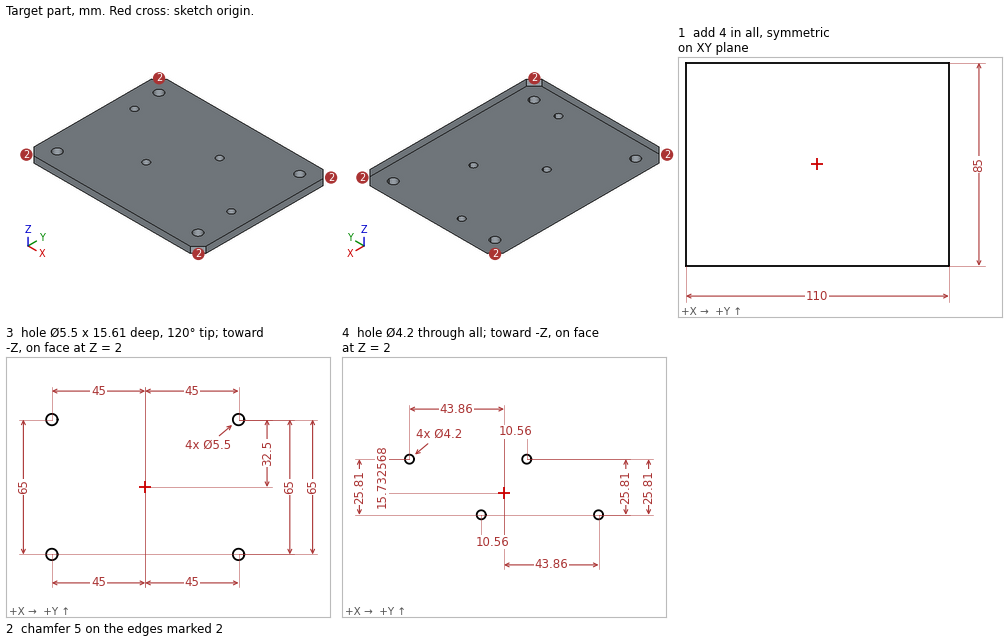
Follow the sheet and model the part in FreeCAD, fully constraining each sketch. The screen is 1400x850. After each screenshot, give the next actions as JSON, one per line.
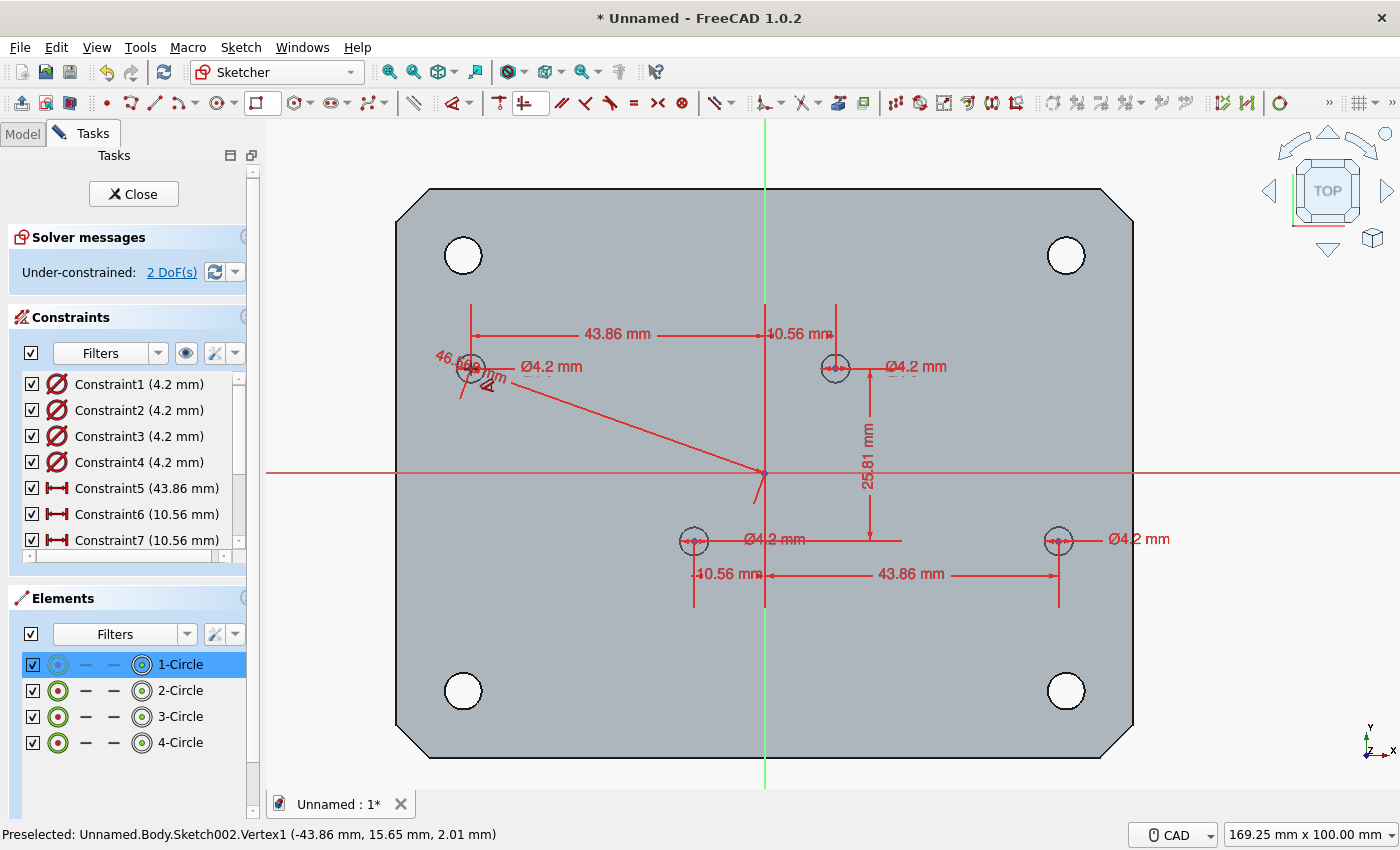
{"action": "left_click", "coordinate": [694, 541]}
{"action": "left_click", "coordinate": [437, 455]}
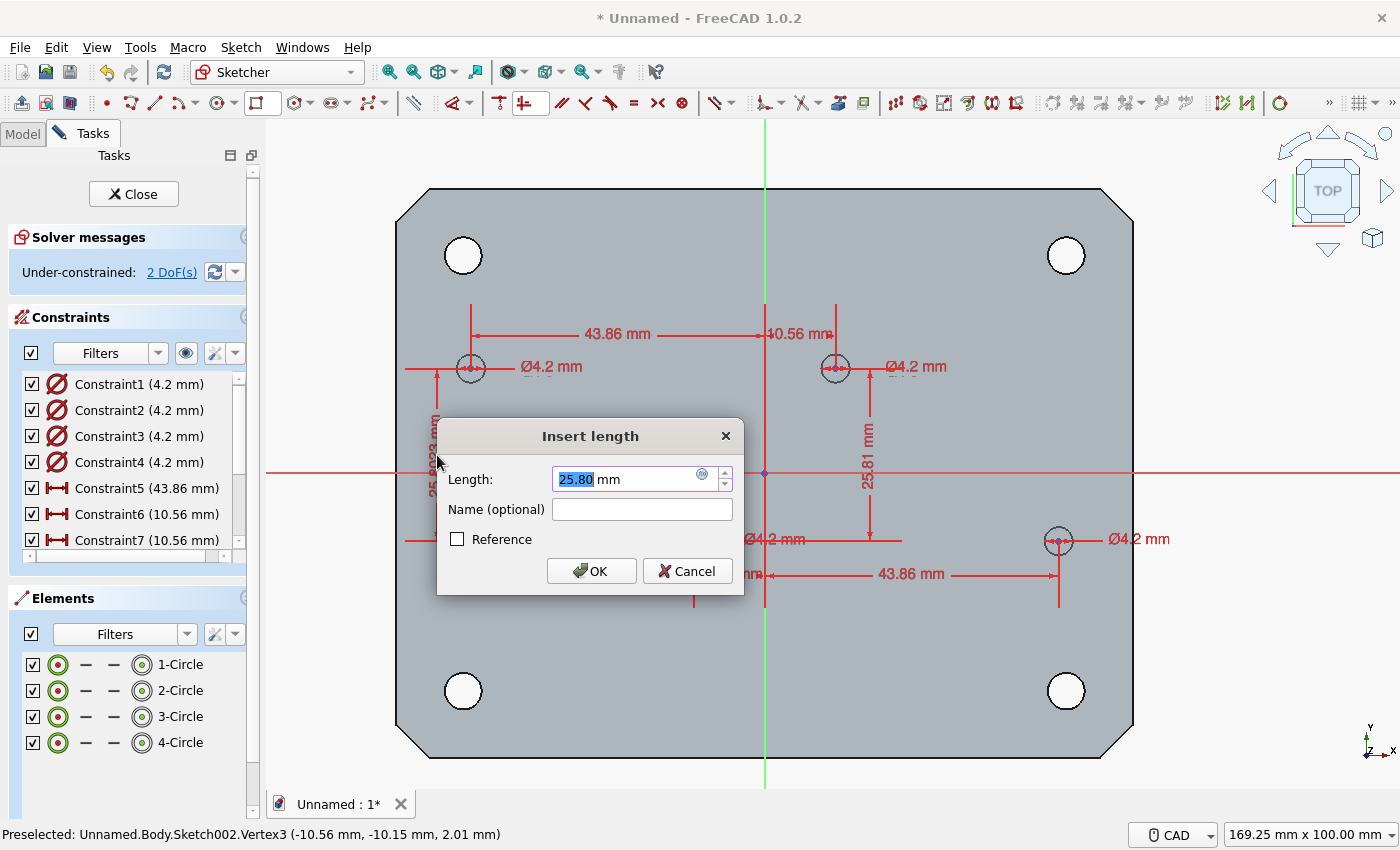
{"action": "type", "text": "25.81"}
{"action": "key", "text": "Return"}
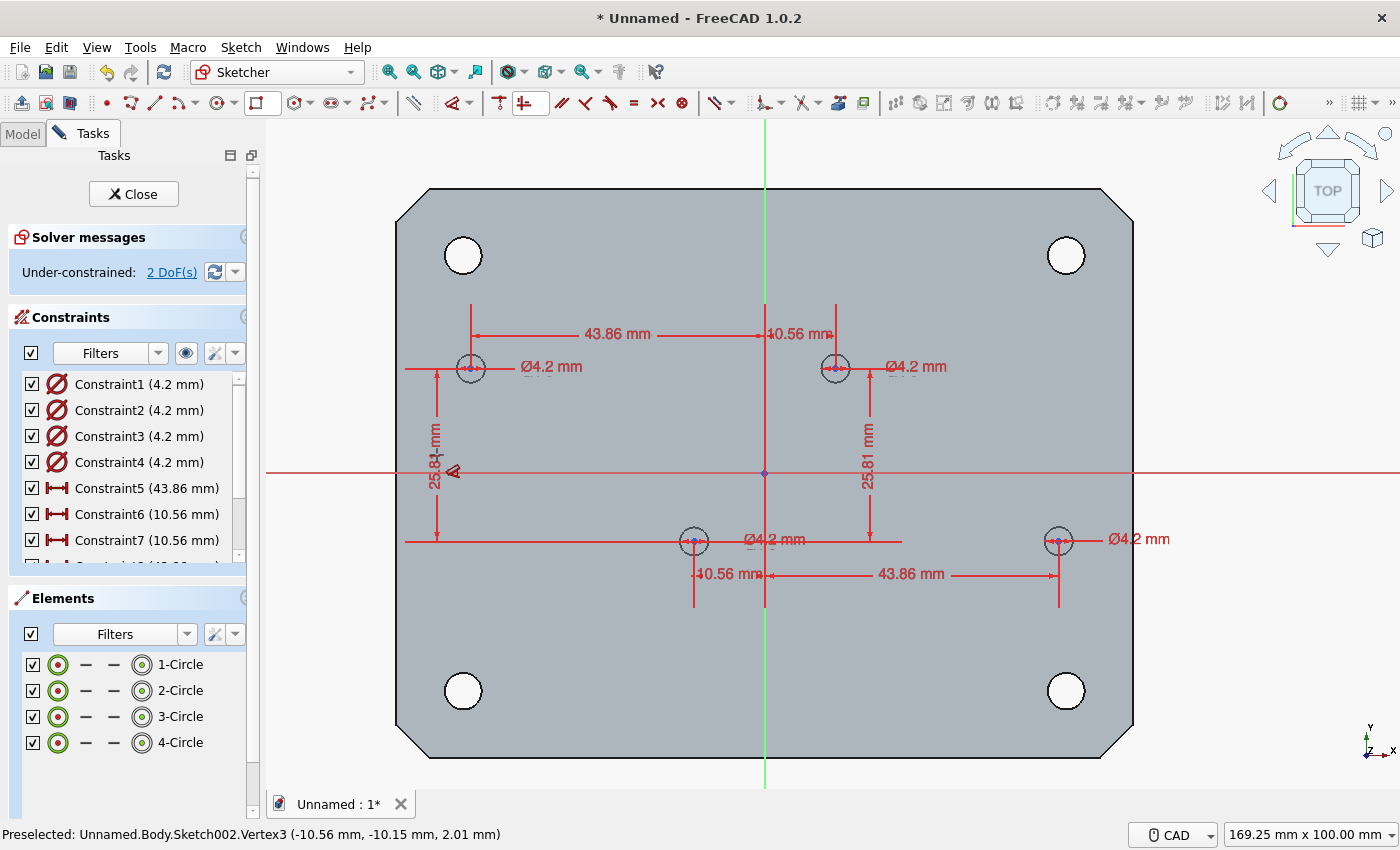
{"action": "left_click", "coordinate": [836, 369]}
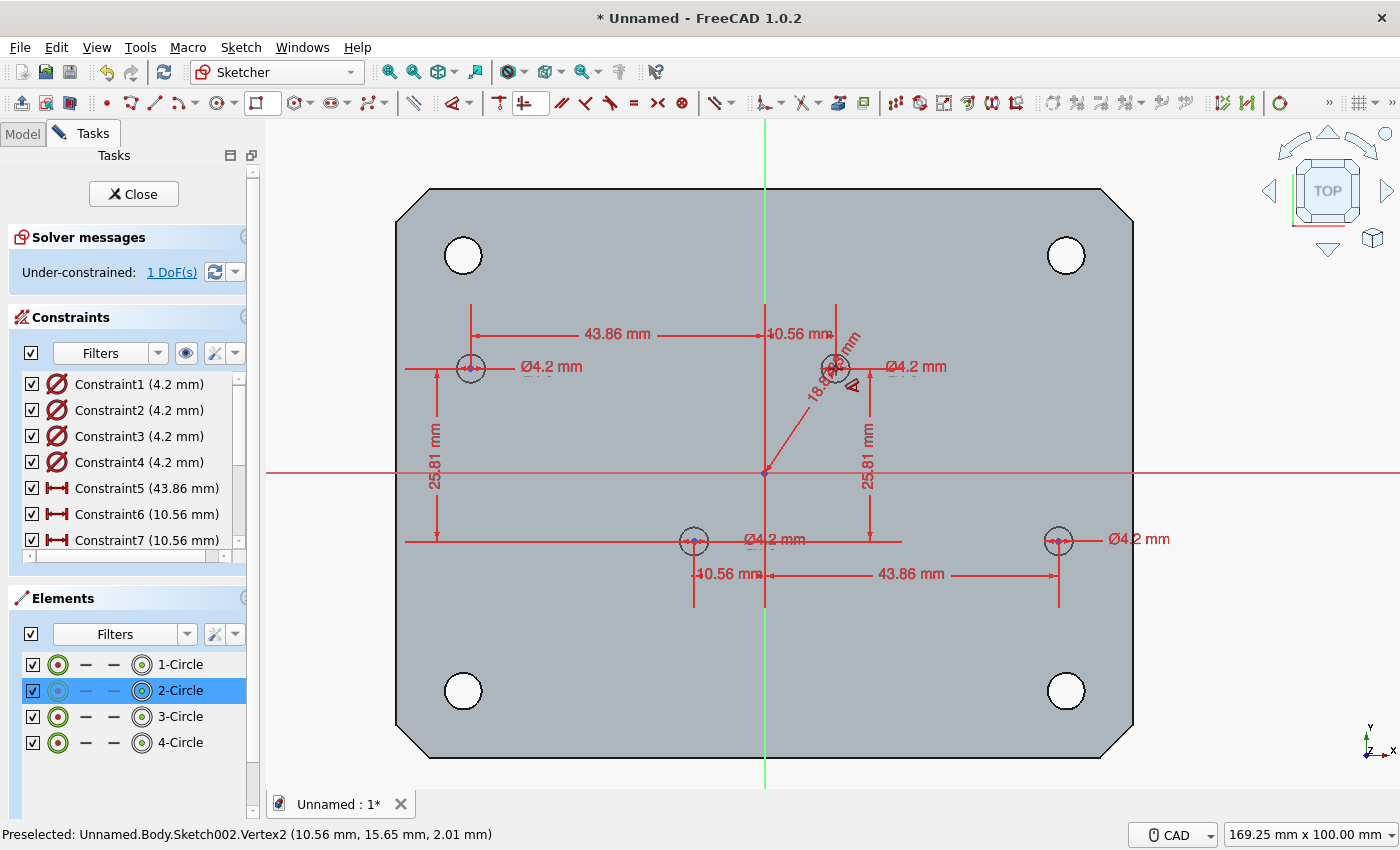
{"action": "left_click", "coordinate": [1059, 541]}
{"action": "left_click", "coordinate": [1093, 455]}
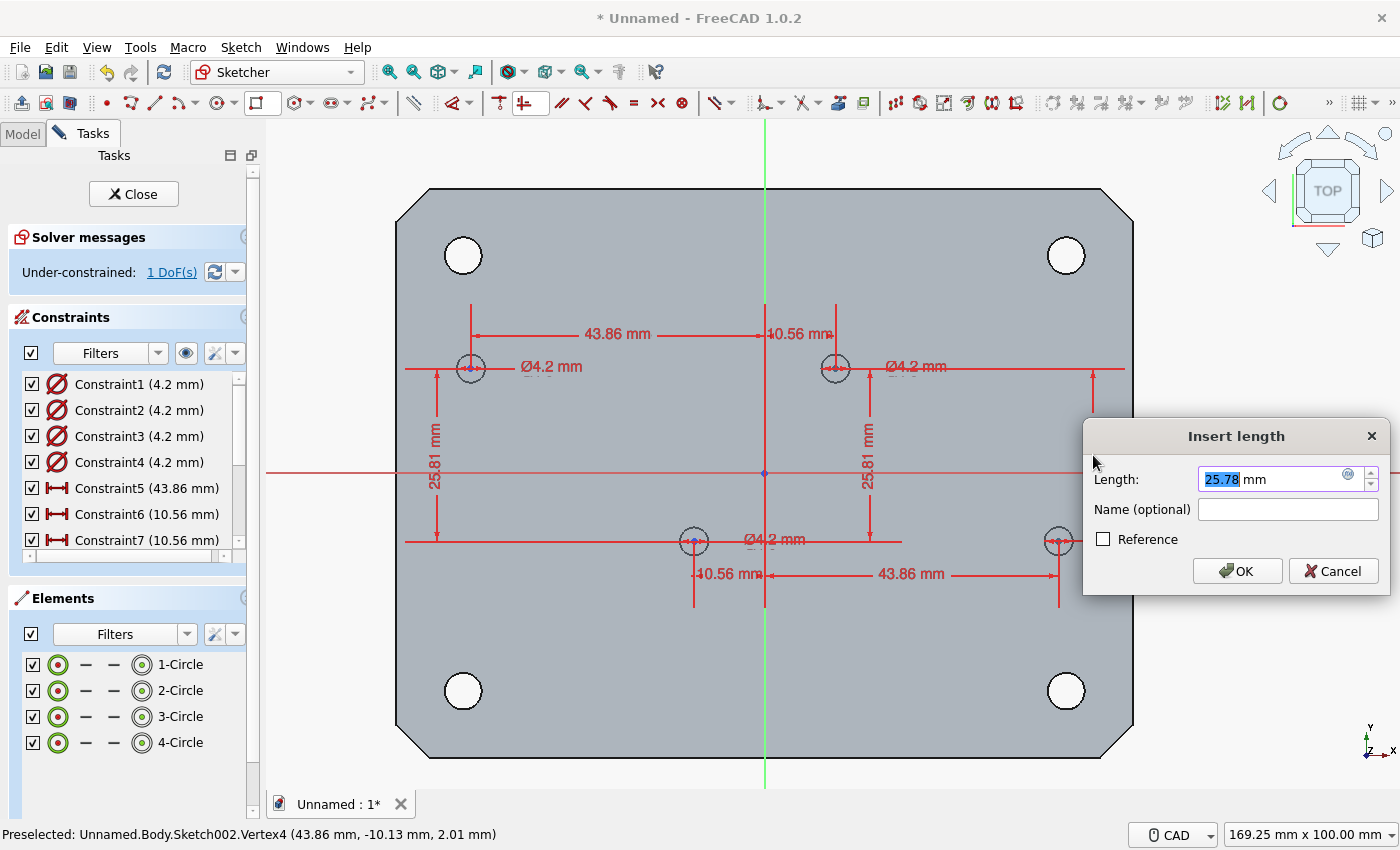
{"action": "type", "text": "25.81"}
{"action": "key", "text": "Return"}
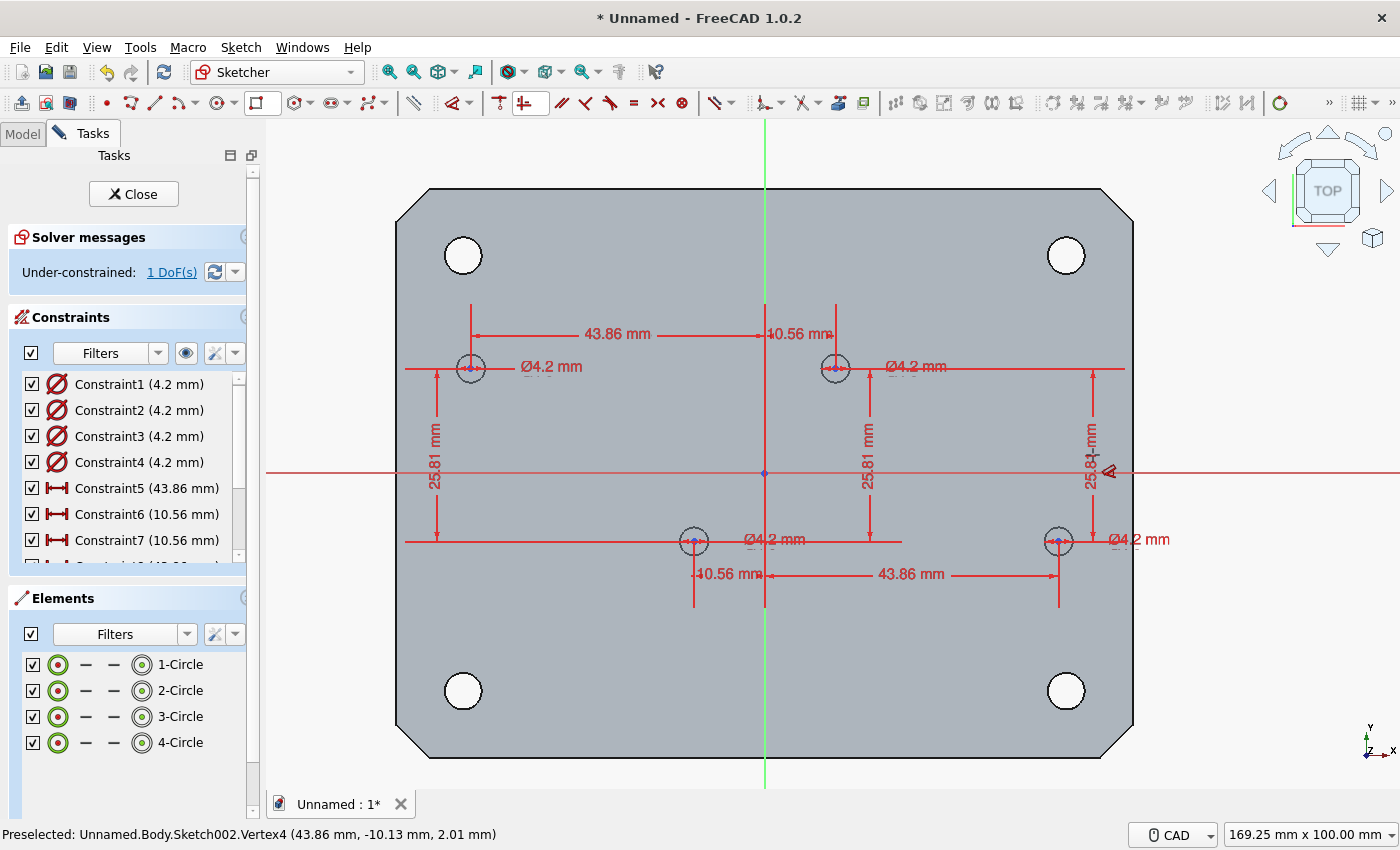
{"action": "left_click", "coordinate": [471, 369]}
{"action": "left_click", "coordinate": [437, 421]}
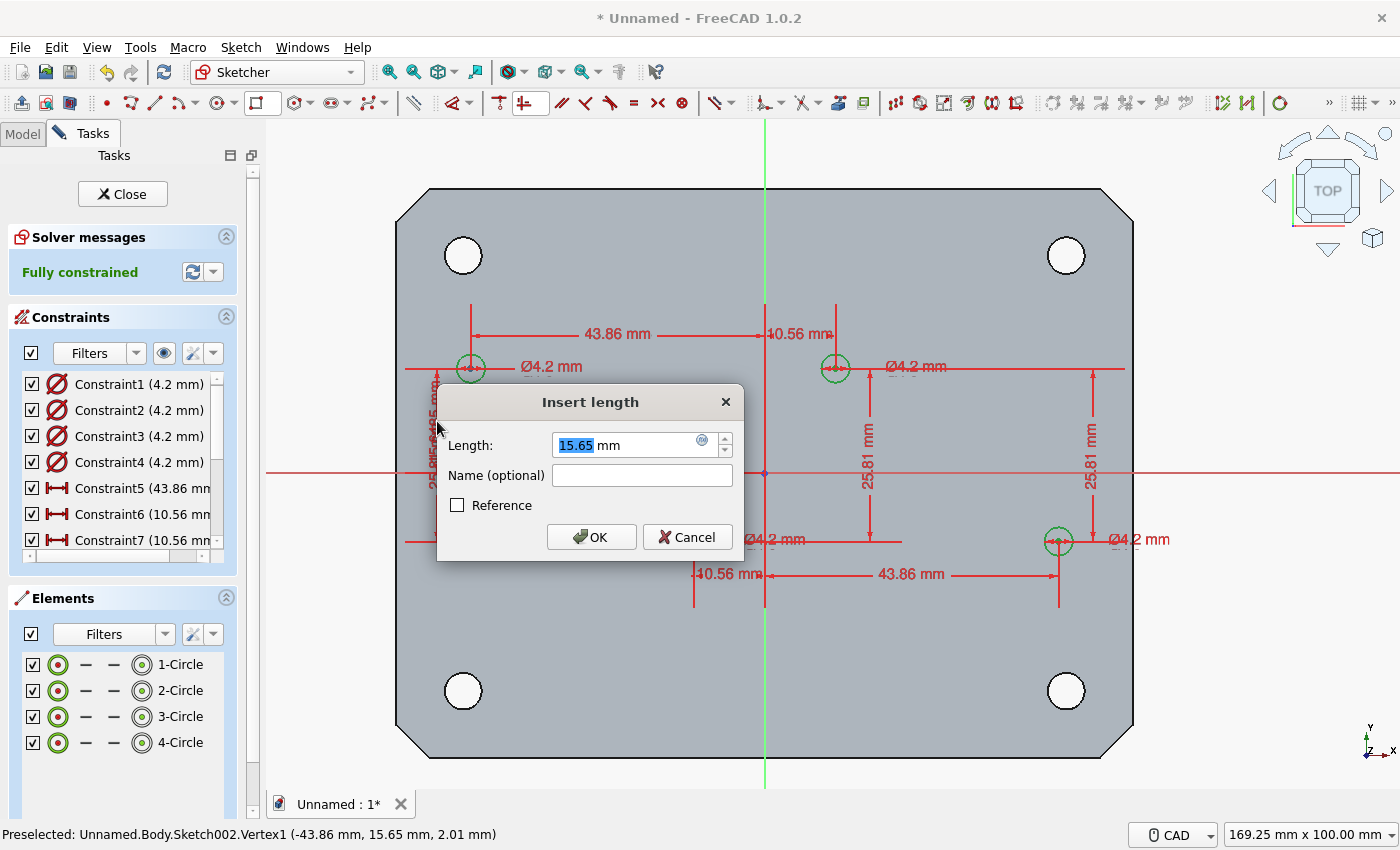
{"action": "type", "text": "15.732568"}
{"action": "key", "text": "Return"}
{"action": "key", "text": "Escape"}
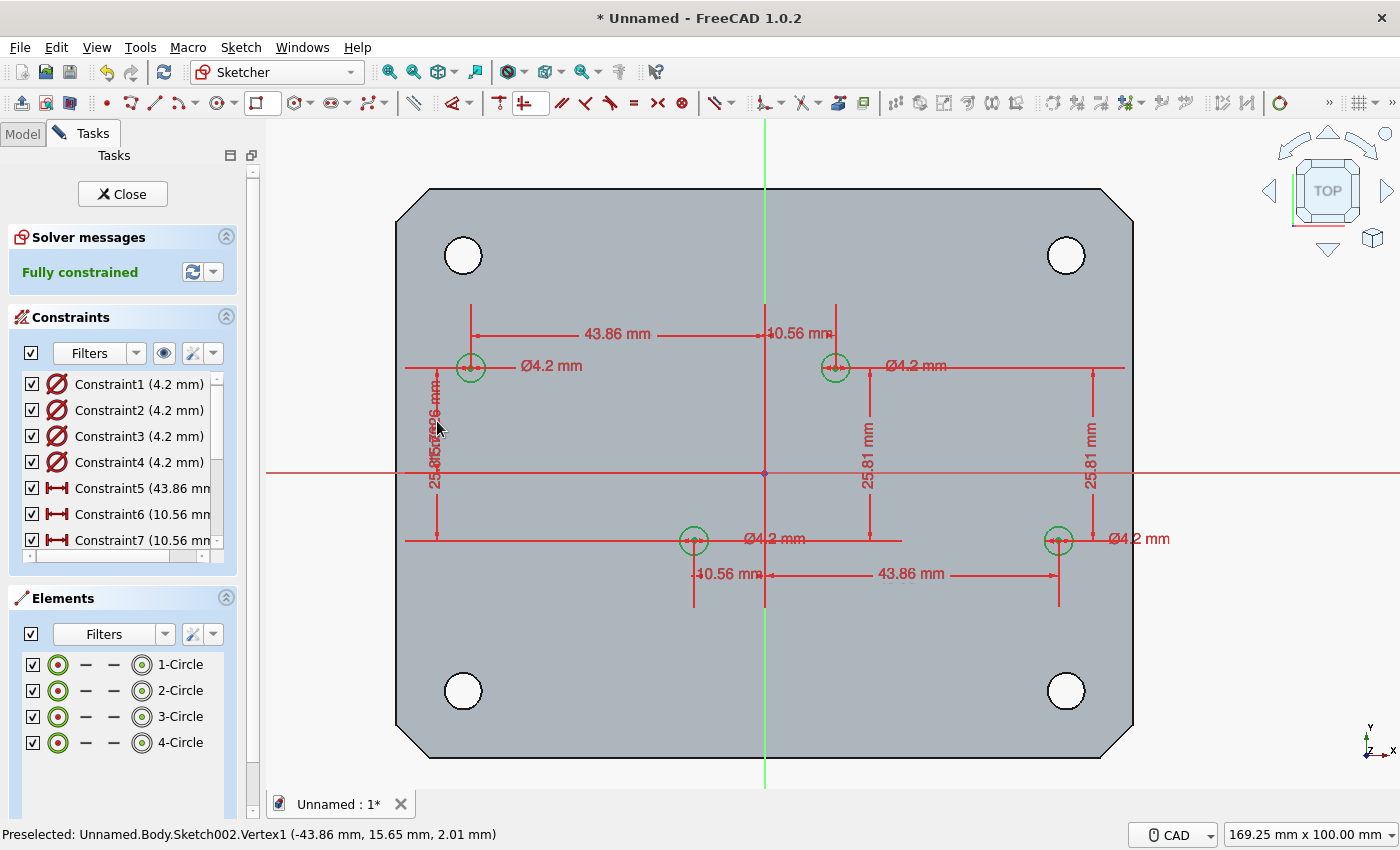
{"action": "left_click", "coordinate": [123, 194]}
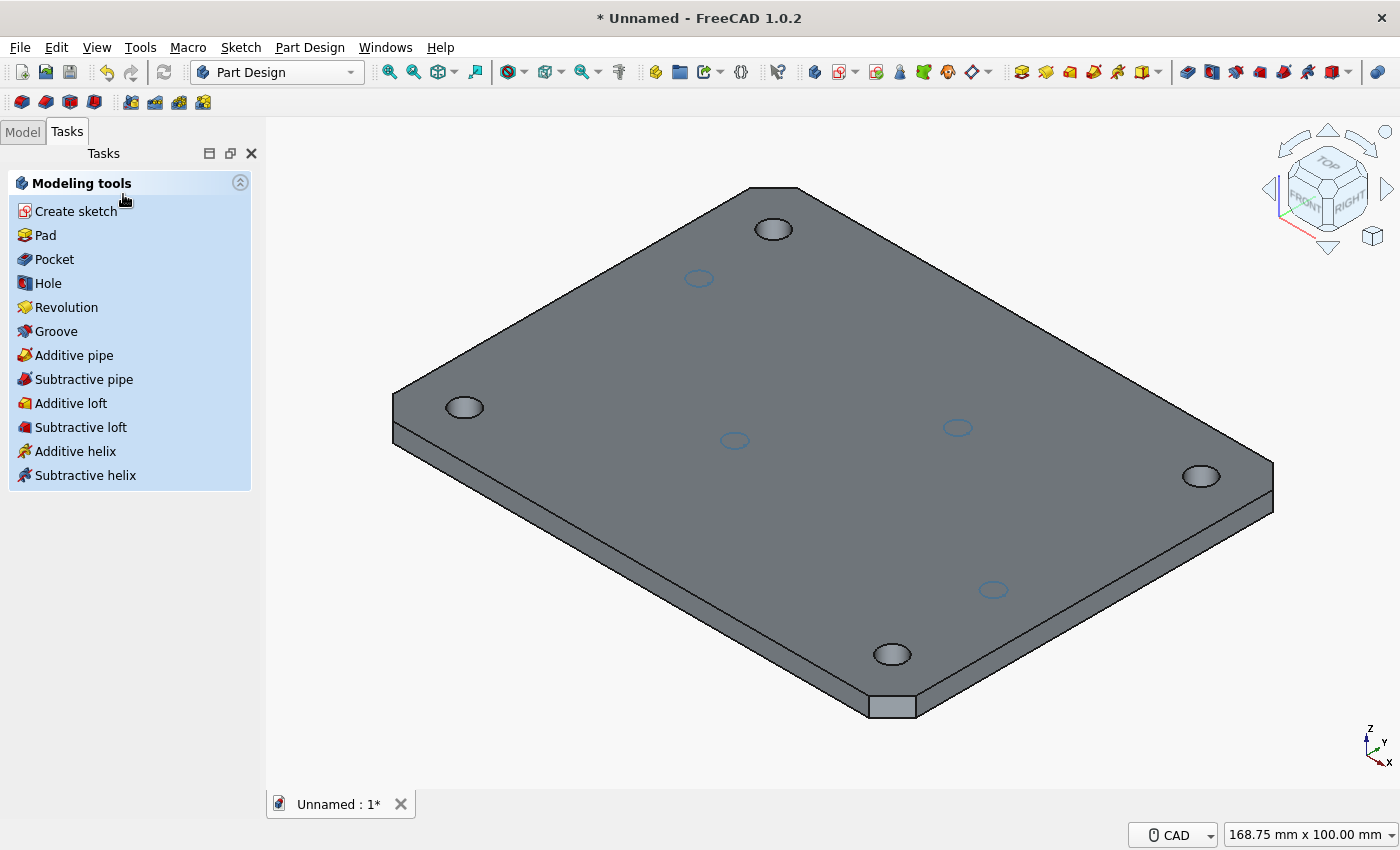
{"action": "left_click", "coordinate": [1212, 72]}